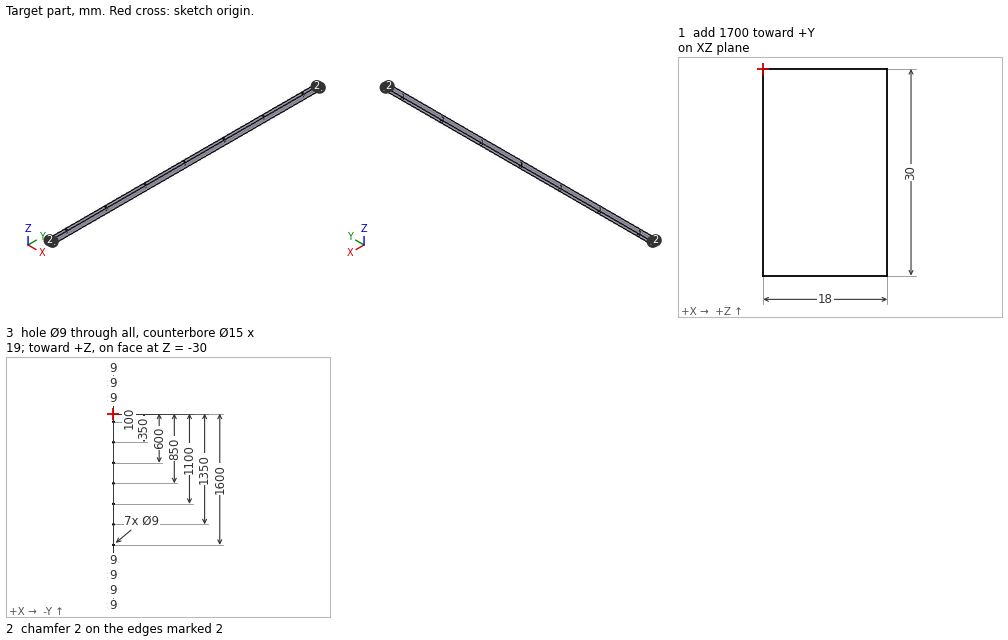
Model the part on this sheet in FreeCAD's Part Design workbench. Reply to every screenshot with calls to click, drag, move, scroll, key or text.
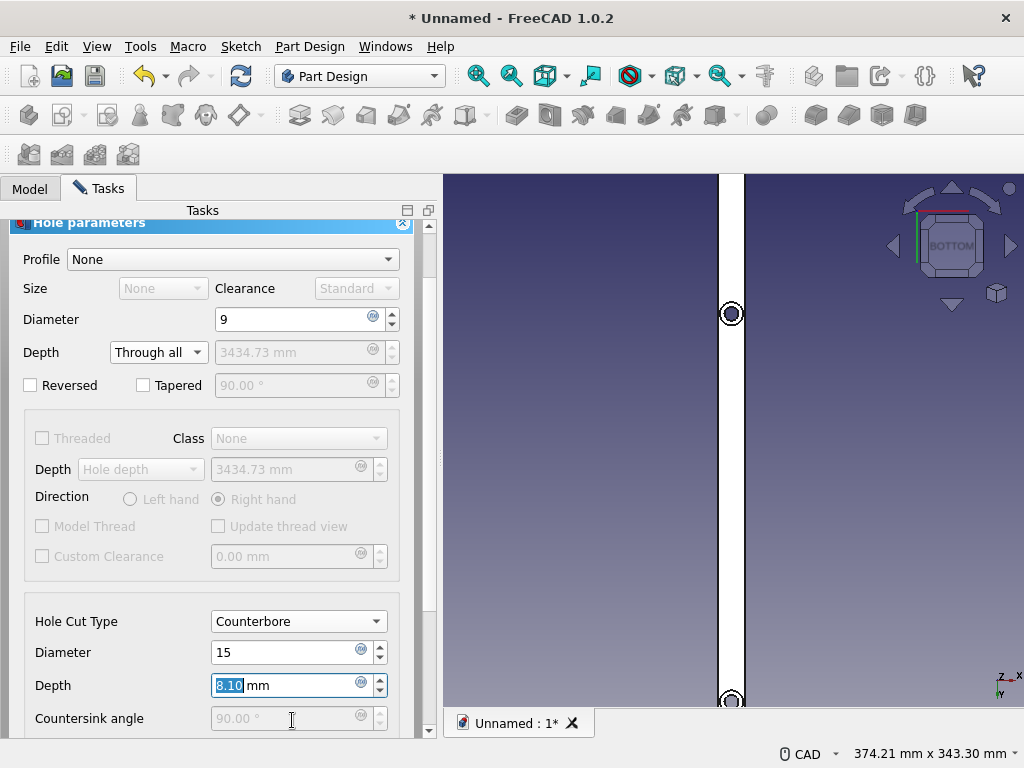
text(19)
key(Tab)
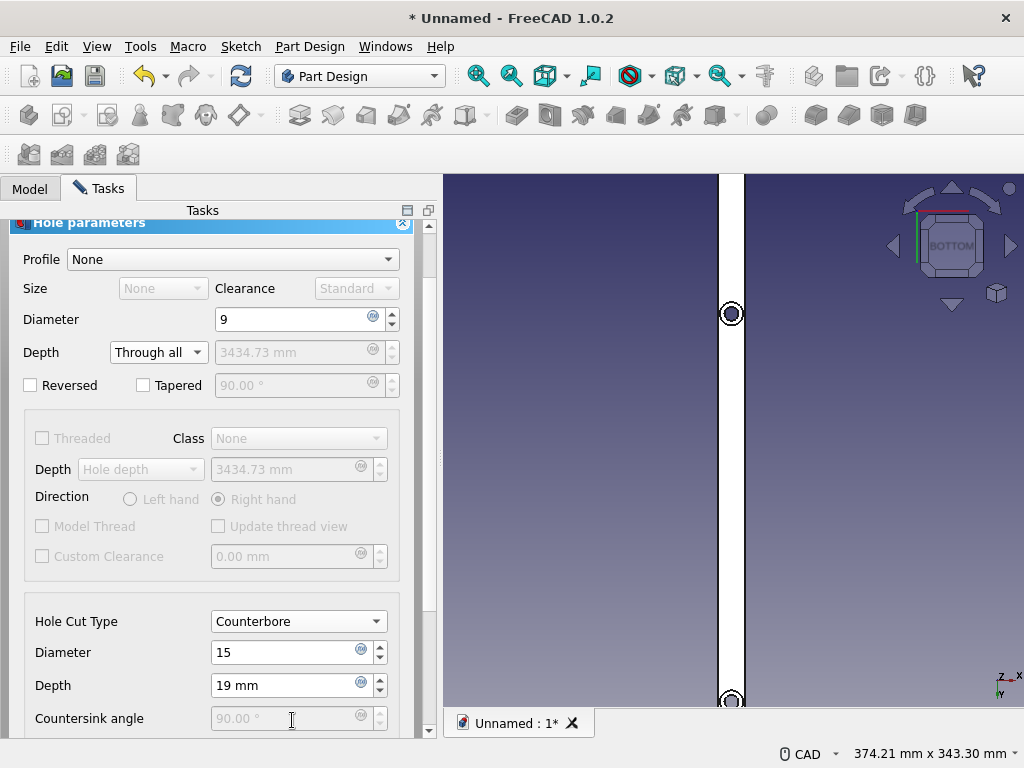
scroll(429, 479, up, 2)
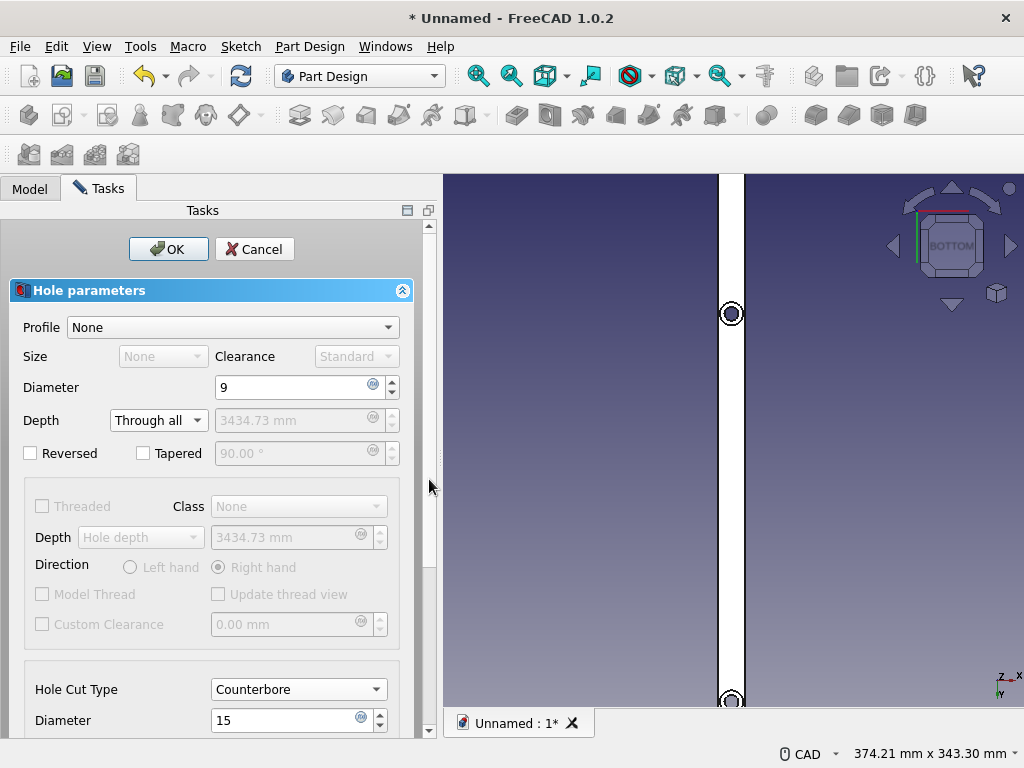
click(169, 249)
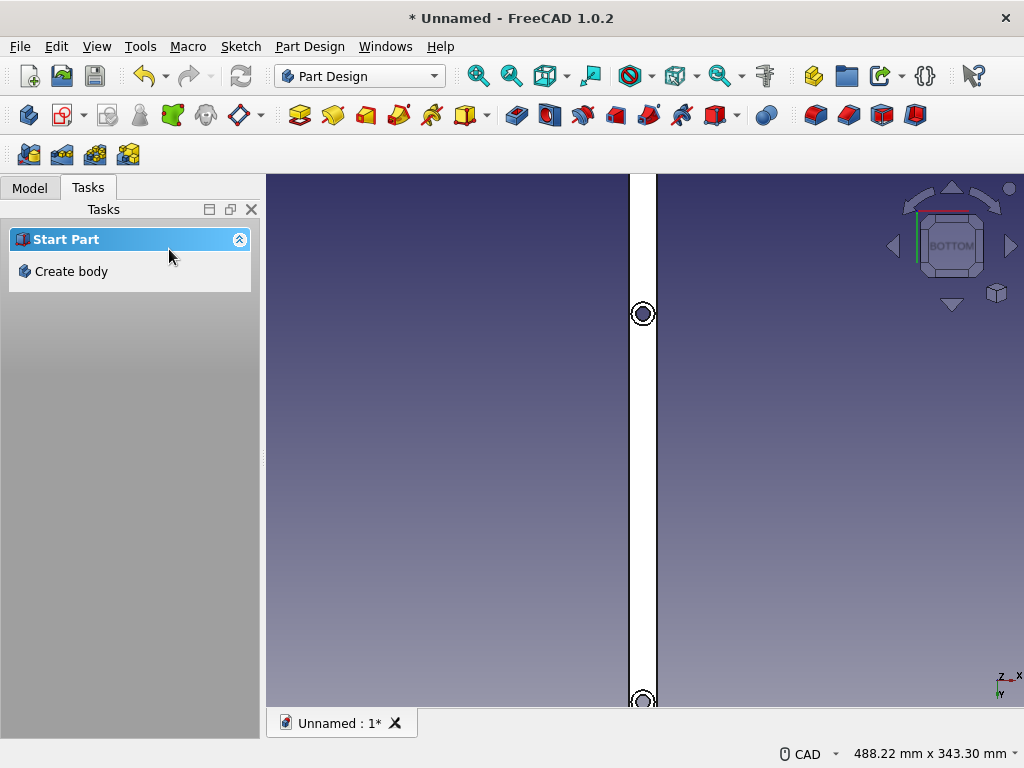
key(0)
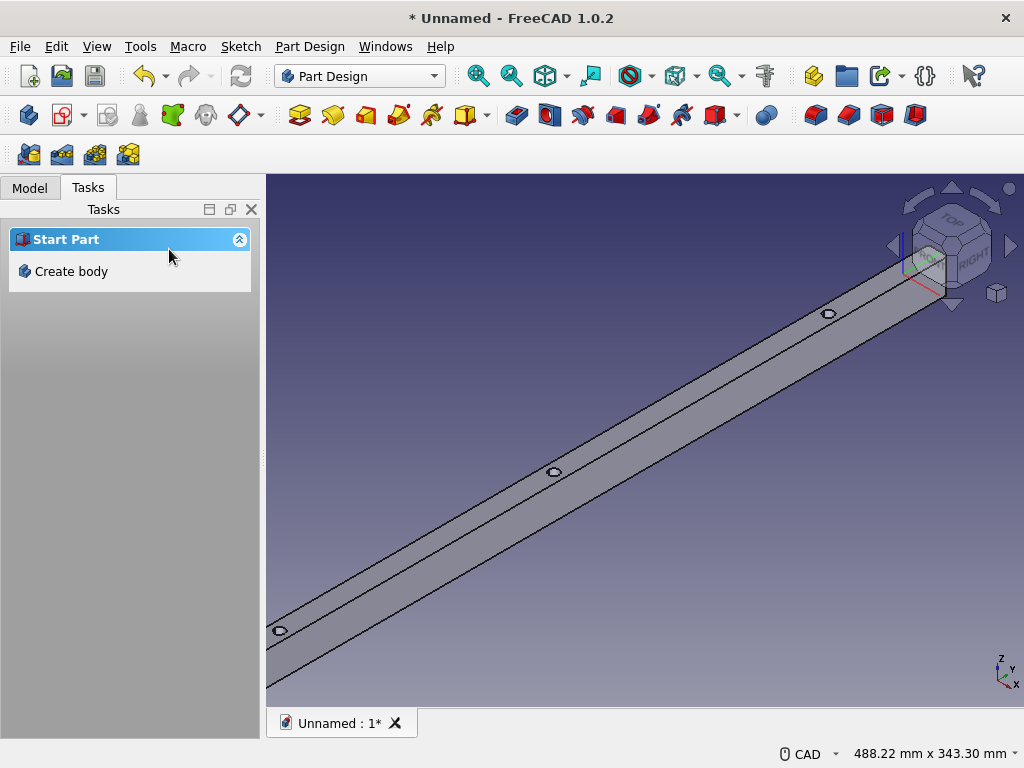
key(v)
key(f)